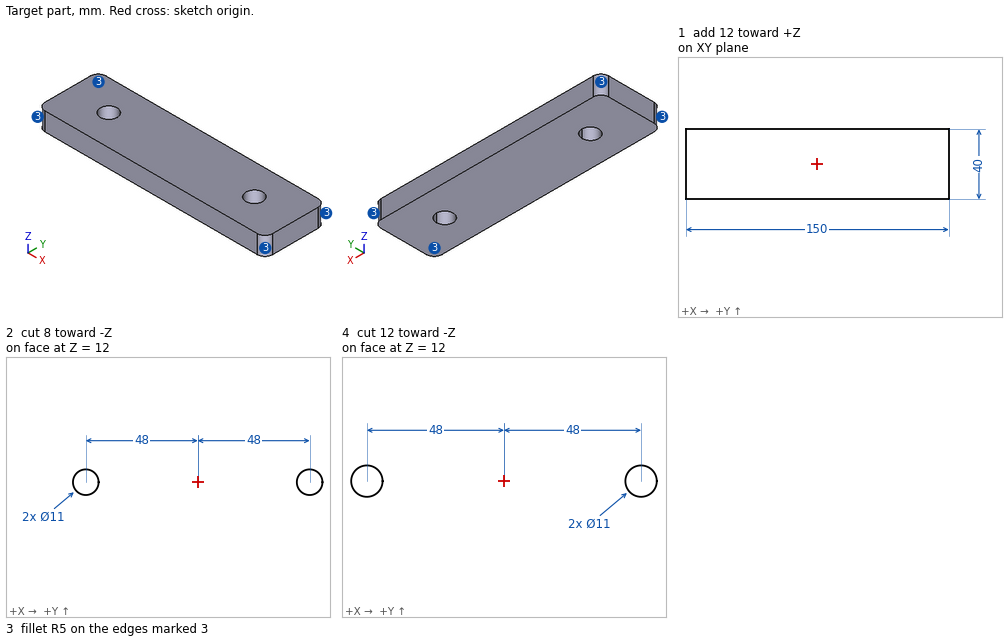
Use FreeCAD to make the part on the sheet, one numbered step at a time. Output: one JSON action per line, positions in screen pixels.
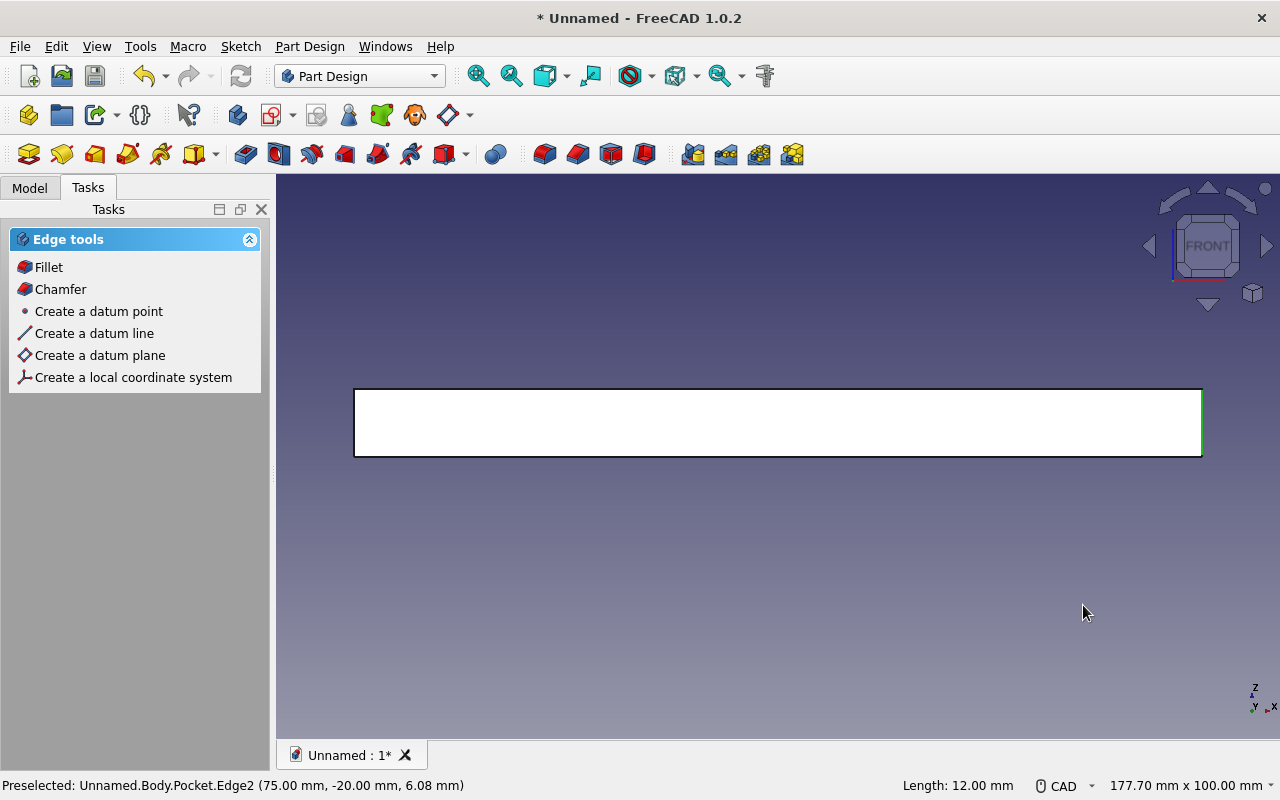
{"action": "left_click", "coordinate": [354, 422], "text": "ctrl"}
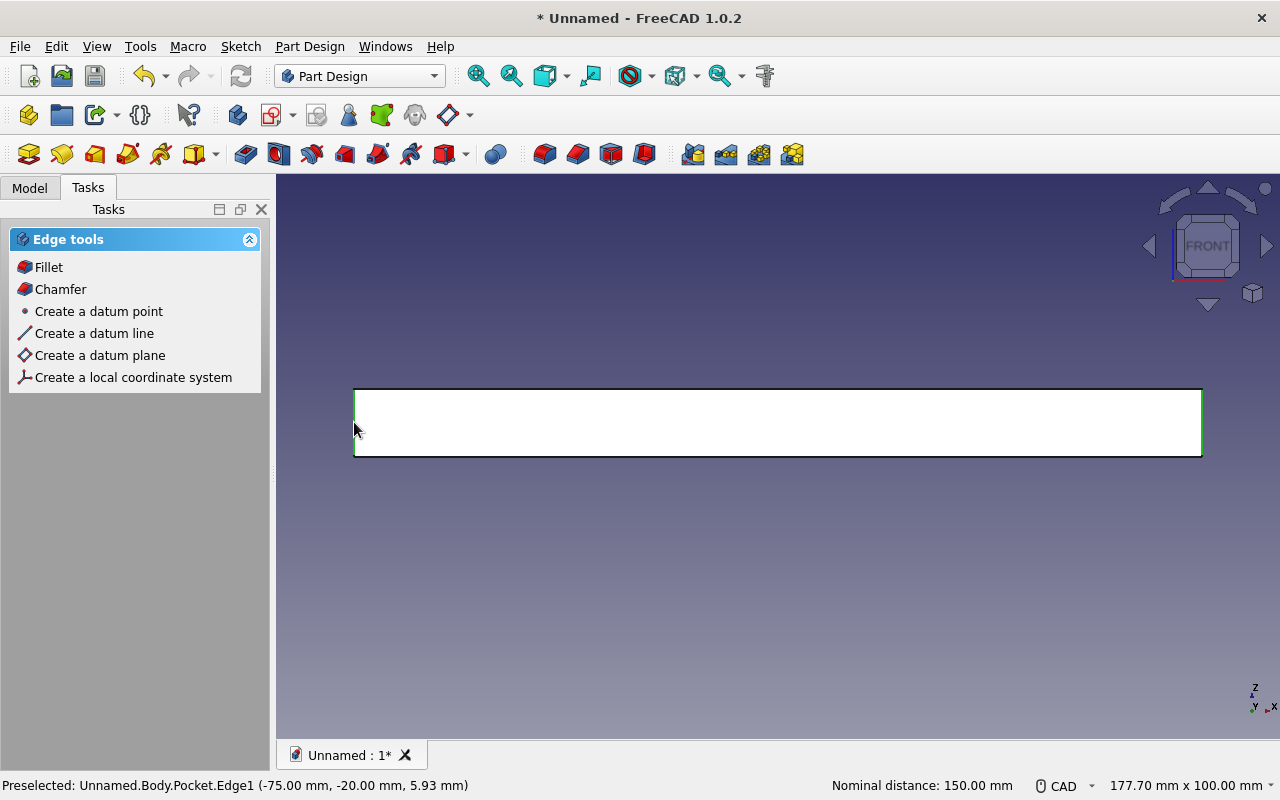
{"action": "key", "text": "3"}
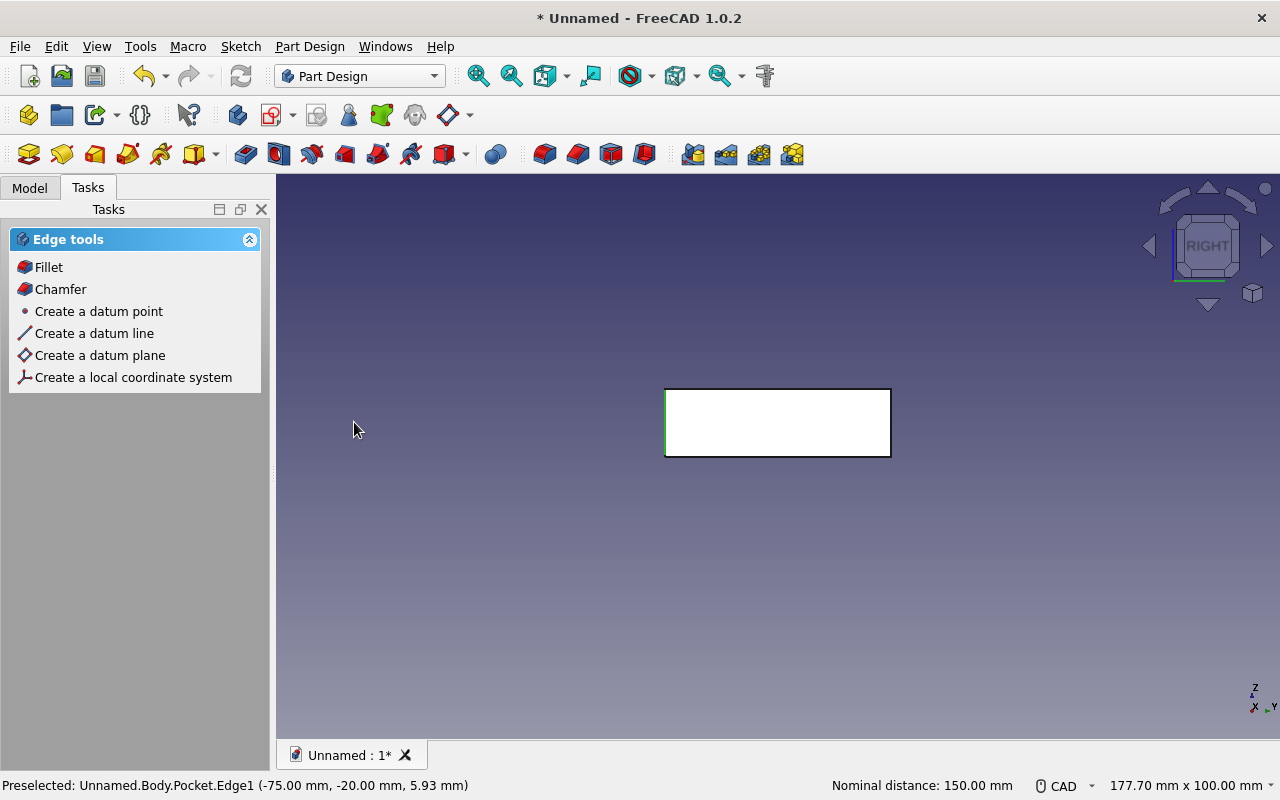
{"action": "left_click", "coordinate": [479, 76]}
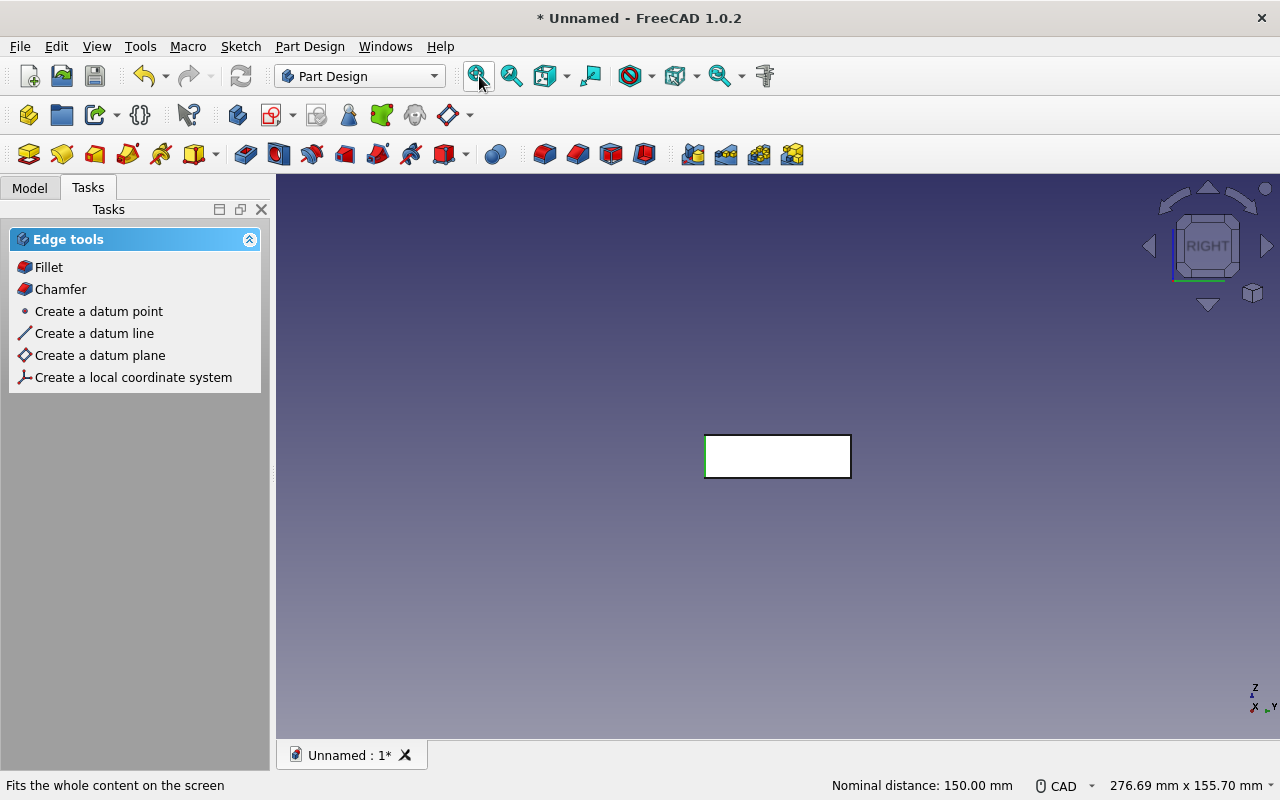
{"action": "left_click", "coordinate": [851, 455], "text": "ctrl"}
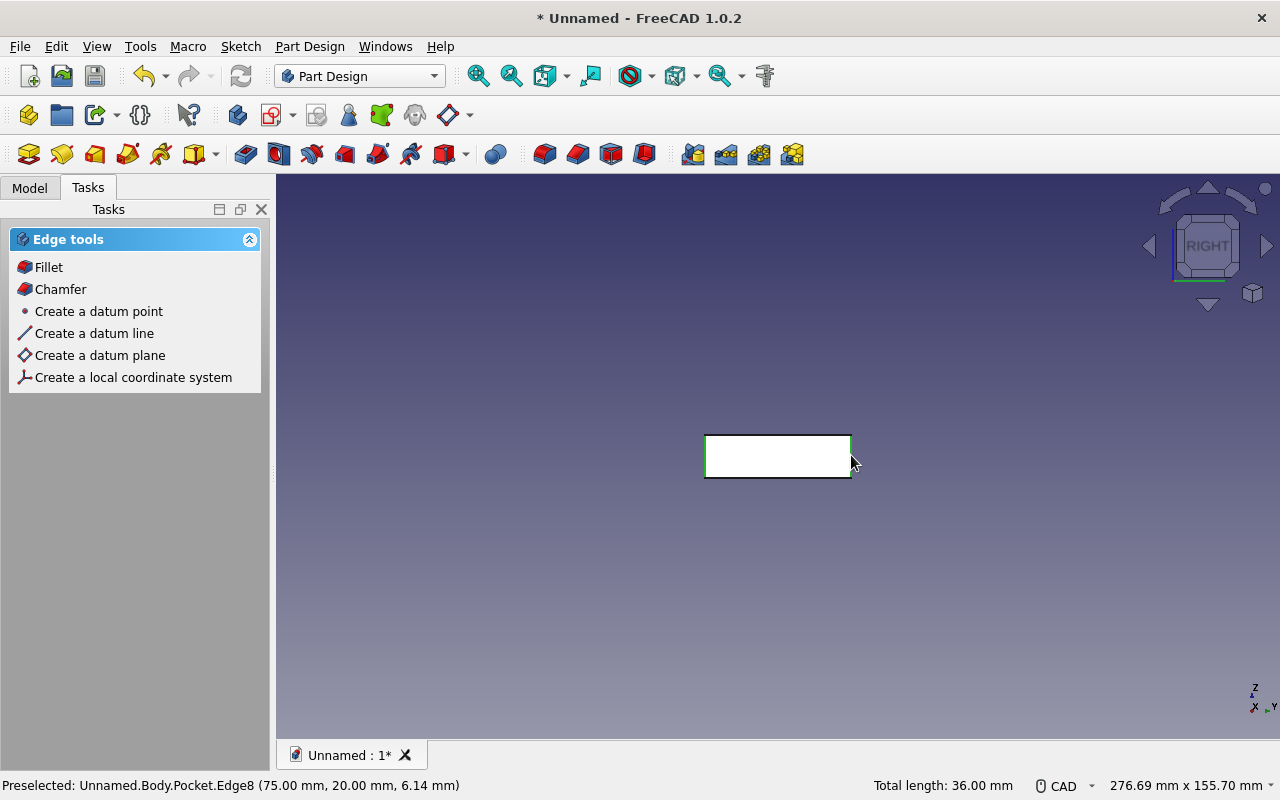
{"action": "key", "text": "5"}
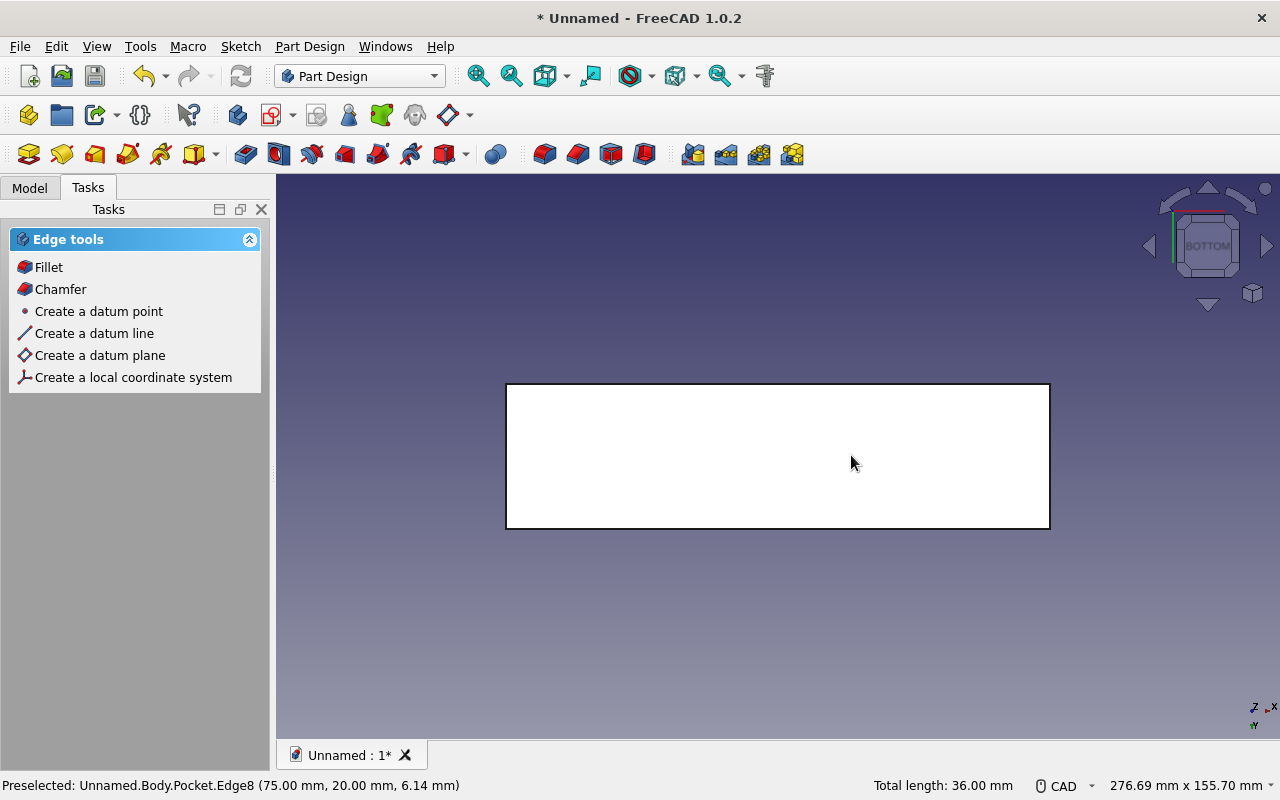
{"action": "key", "text": "4"}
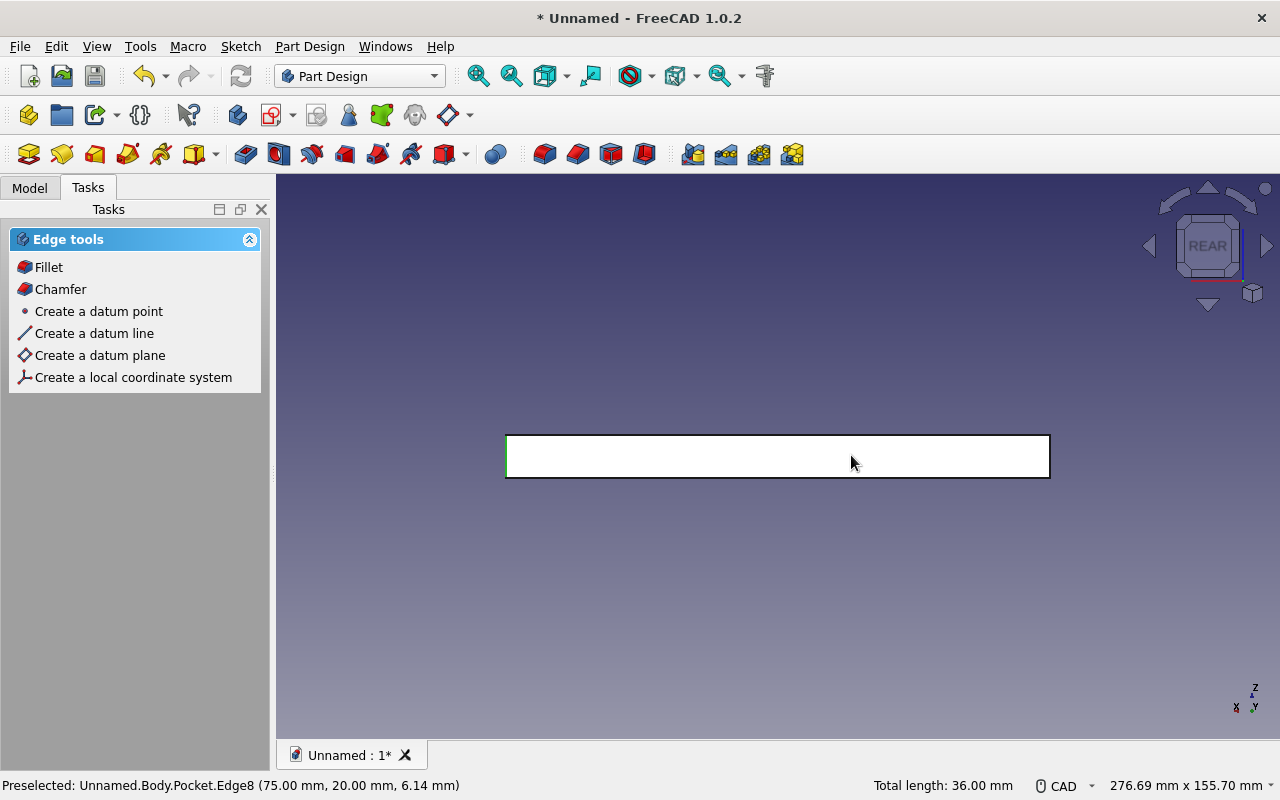
{"action": "left_click", "coordinate": [1050, 455], "text": "ctrl"}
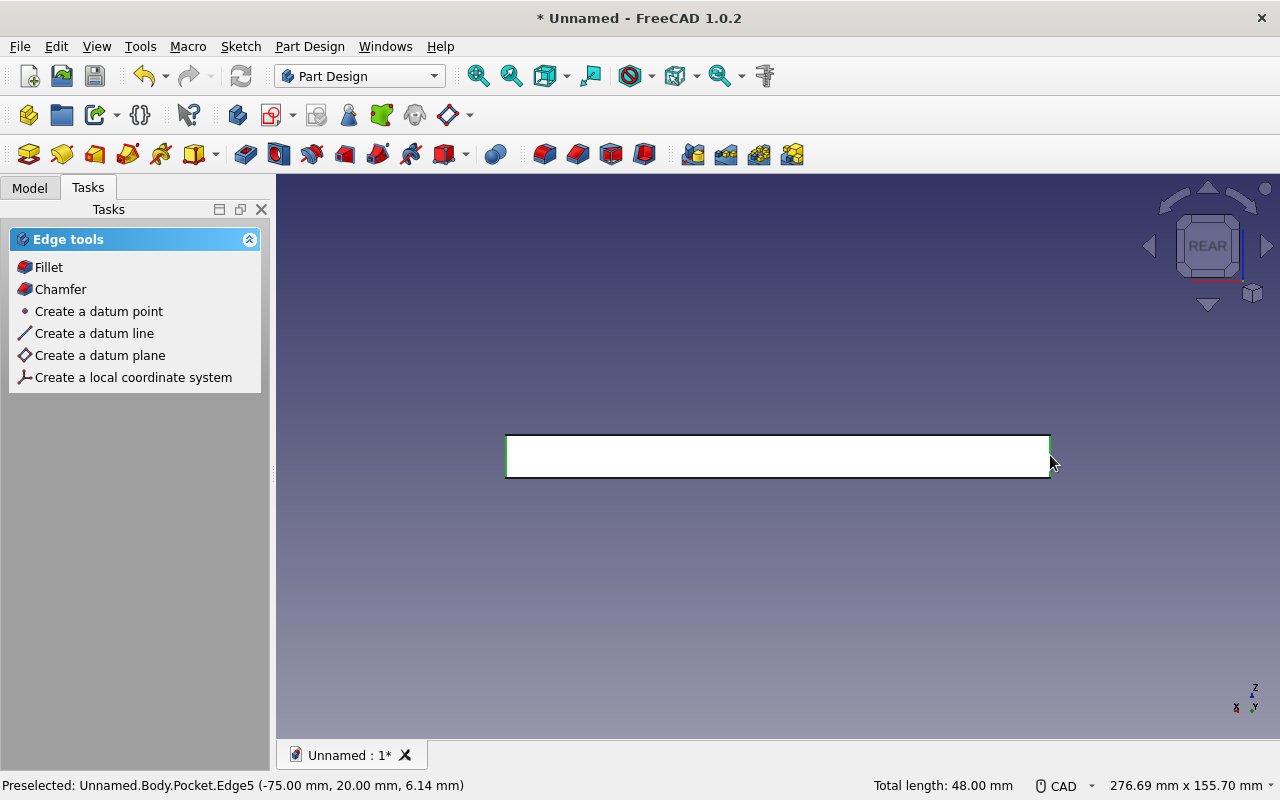
{"action": "left_click", "coordinate": [545, 154]}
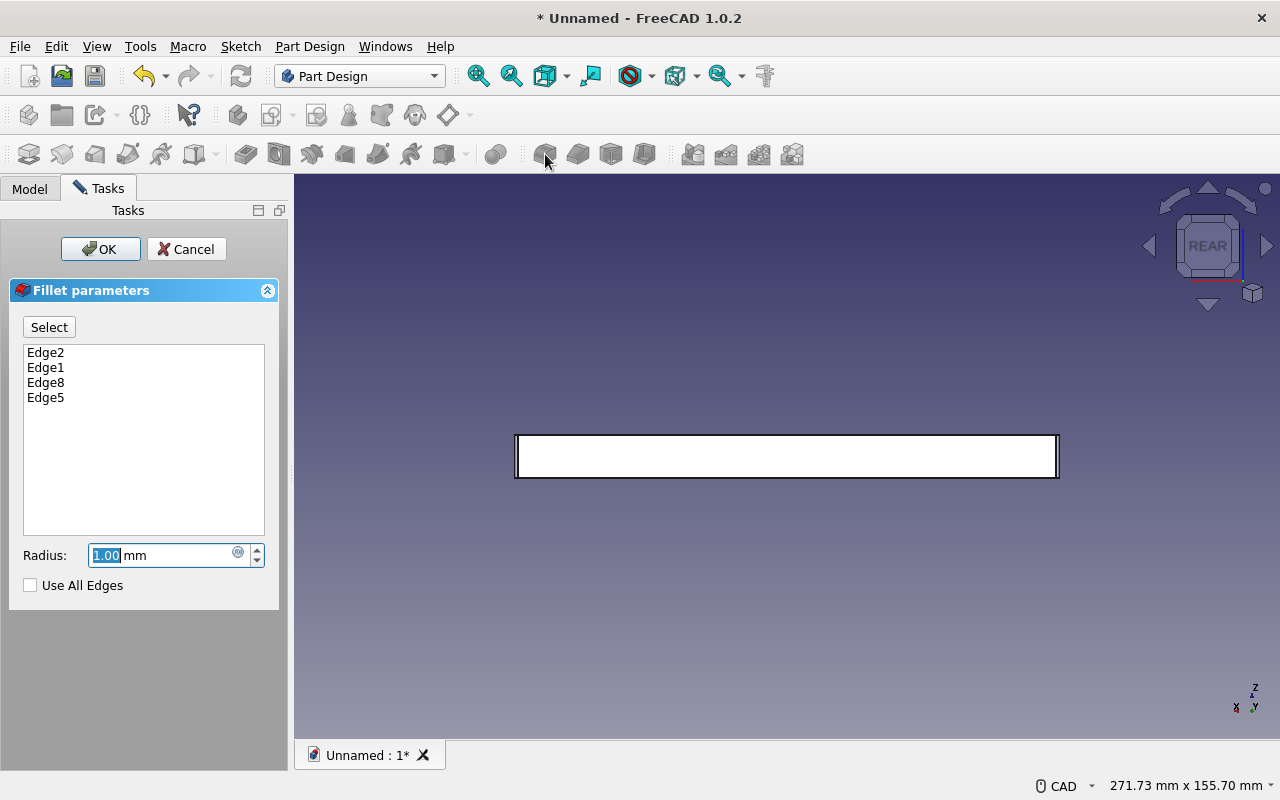
{"action": "type", "text": "5"}
{"action": "key", "text": "Tab"}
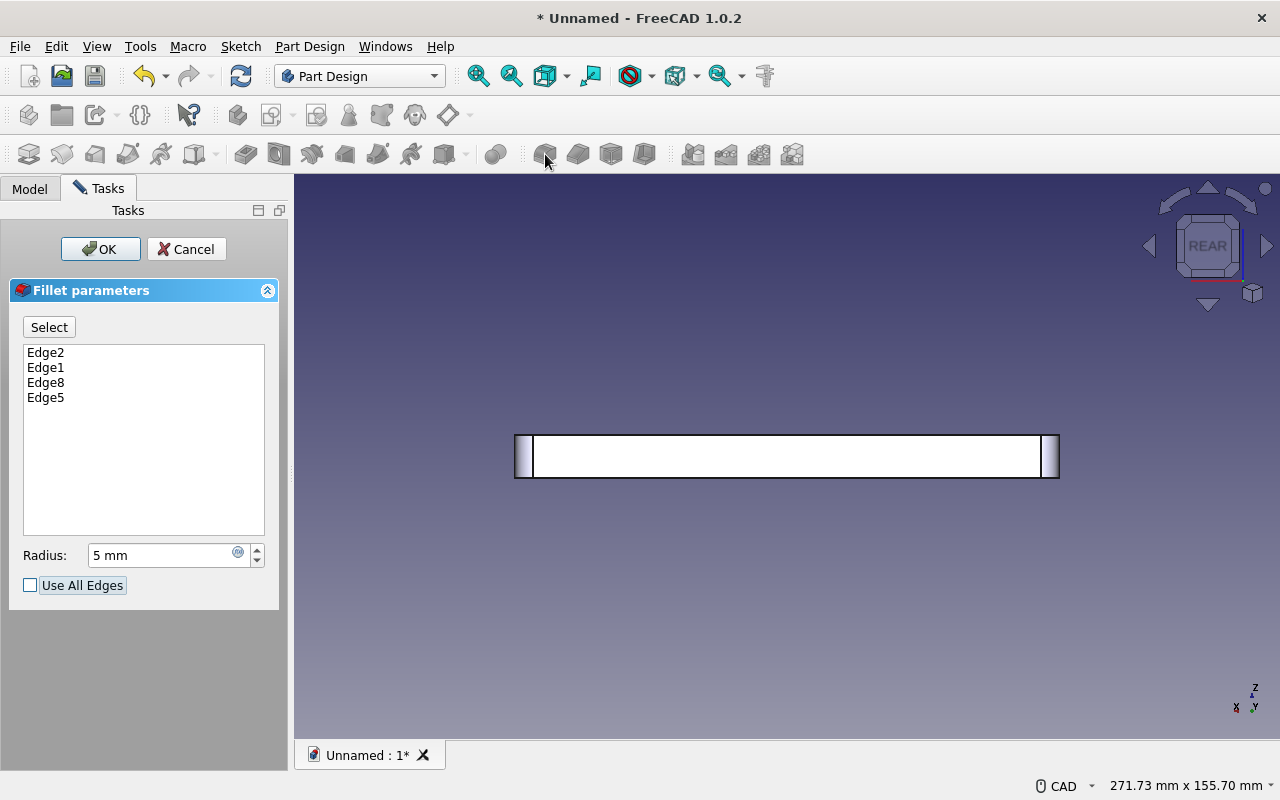
{"action": "left_click", "coordinate": [101, 249]}